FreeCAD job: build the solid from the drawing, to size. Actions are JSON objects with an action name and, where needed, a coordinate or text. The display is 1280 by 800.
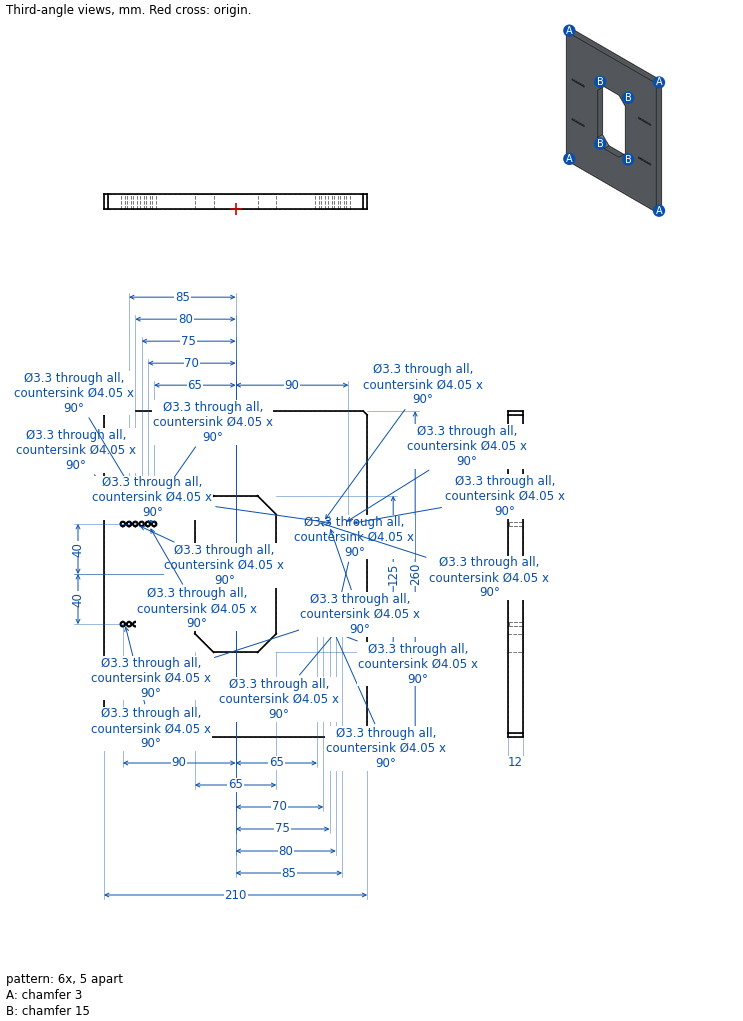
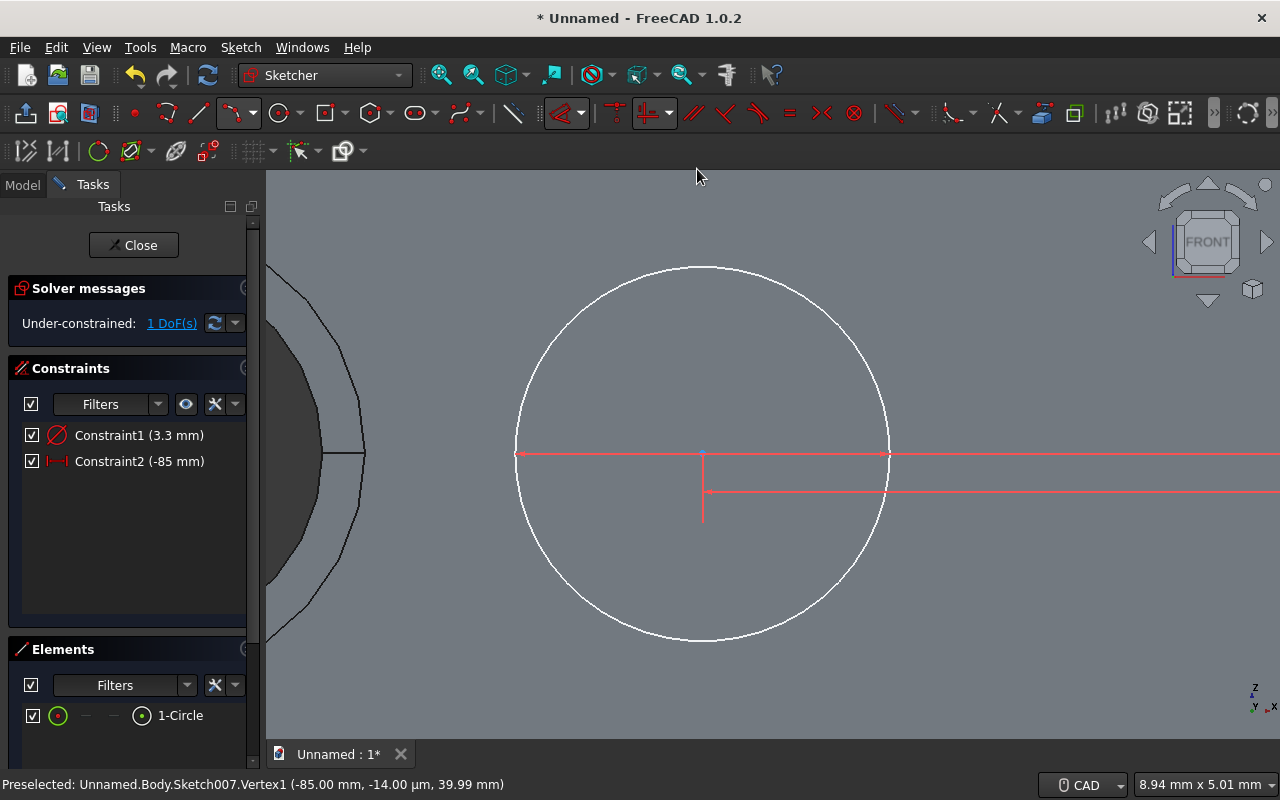
{"action": "left_click", "coordinate": [703, 454]}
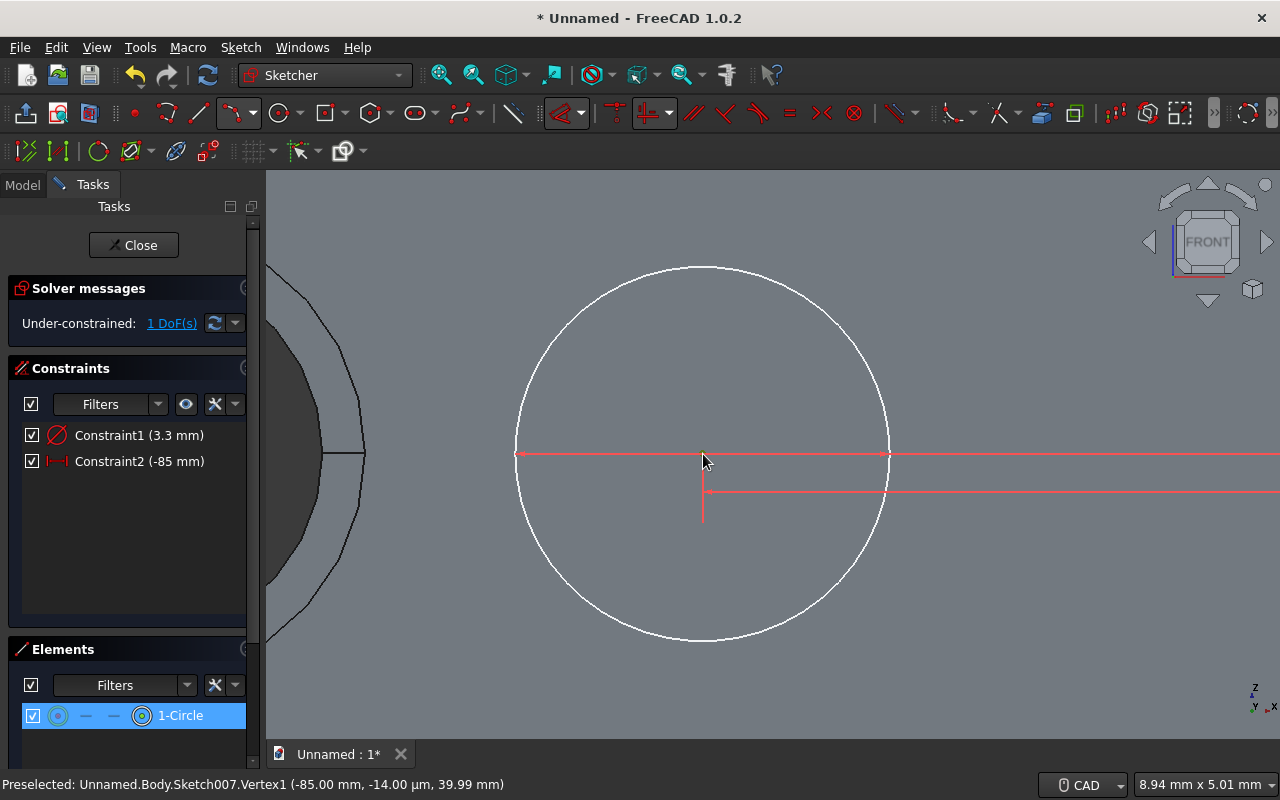
{"action": "key", "text": "i"}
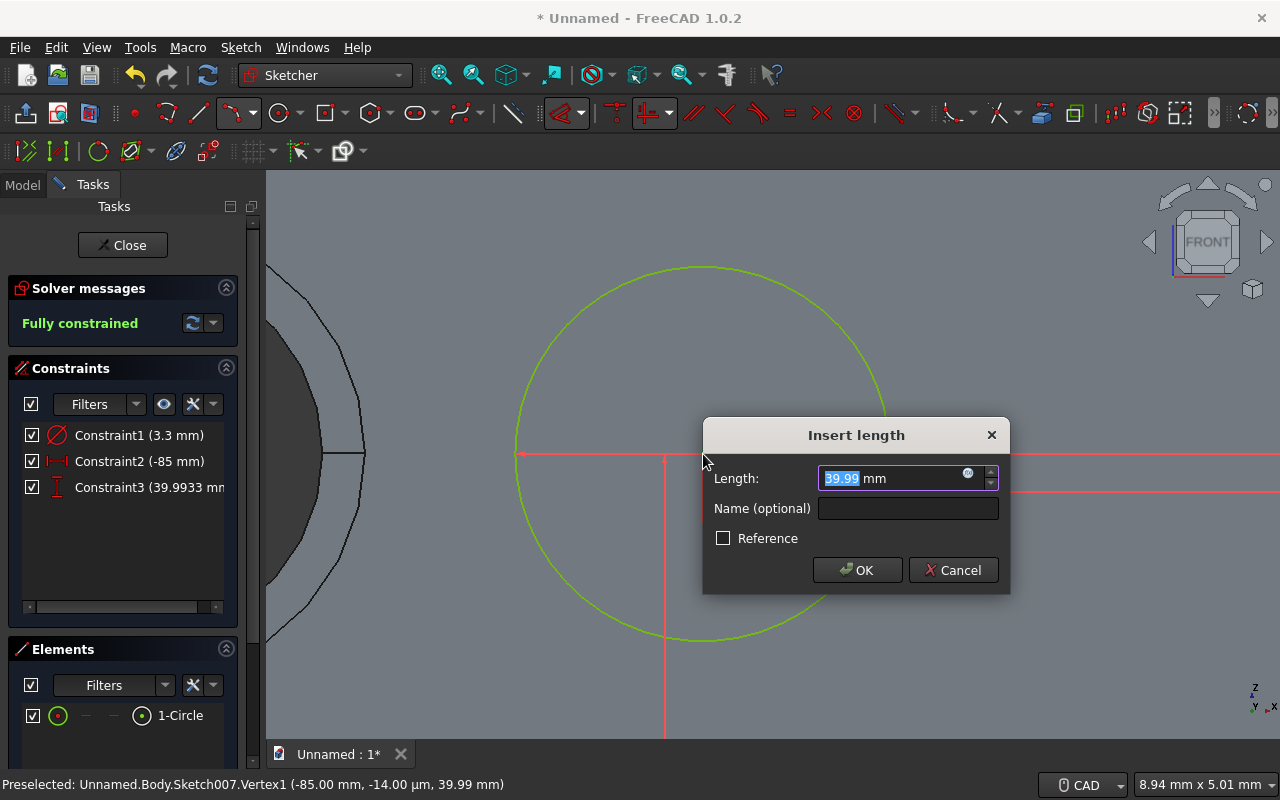
{"action": "type", "text": "40"}
{"action": "key", "text": "Return"}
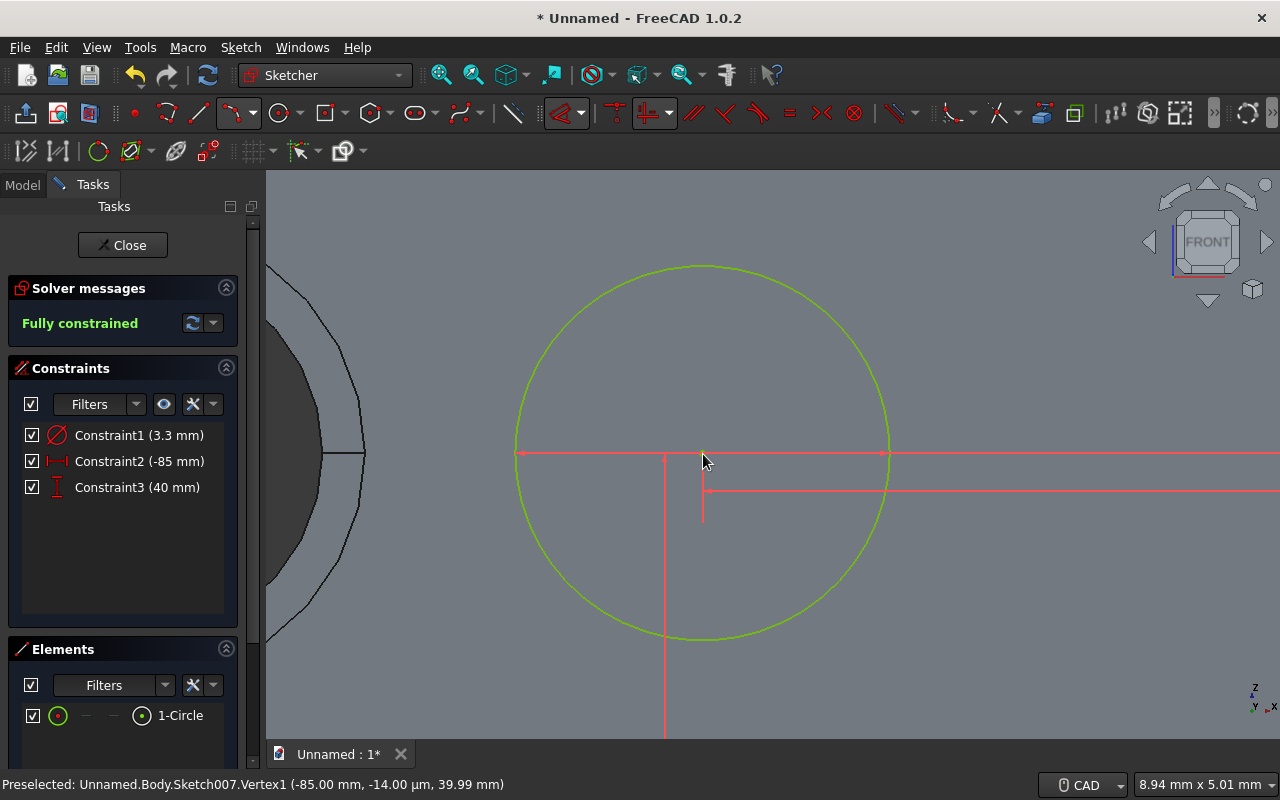
{"action": "left_click", "coordinate": [123, 245]}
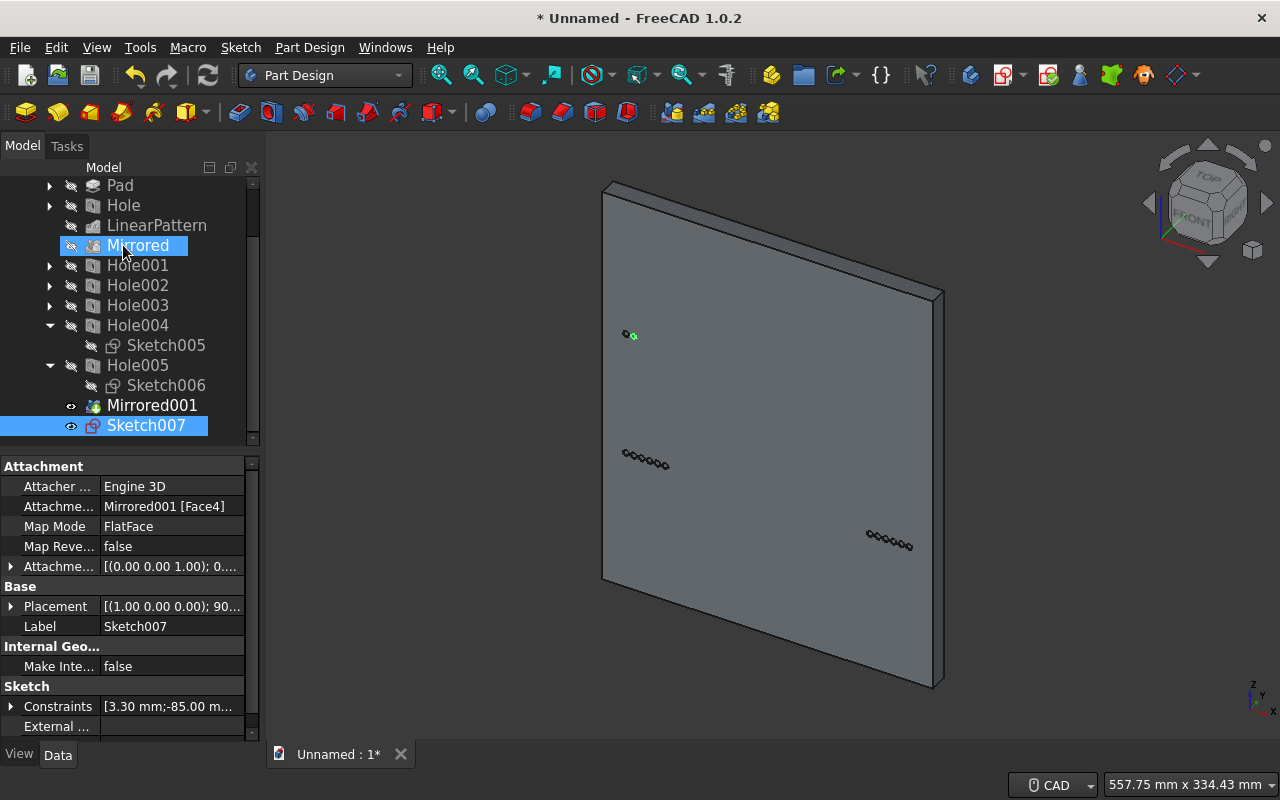
{"action": "left_click", "coordinate": [272, 112]}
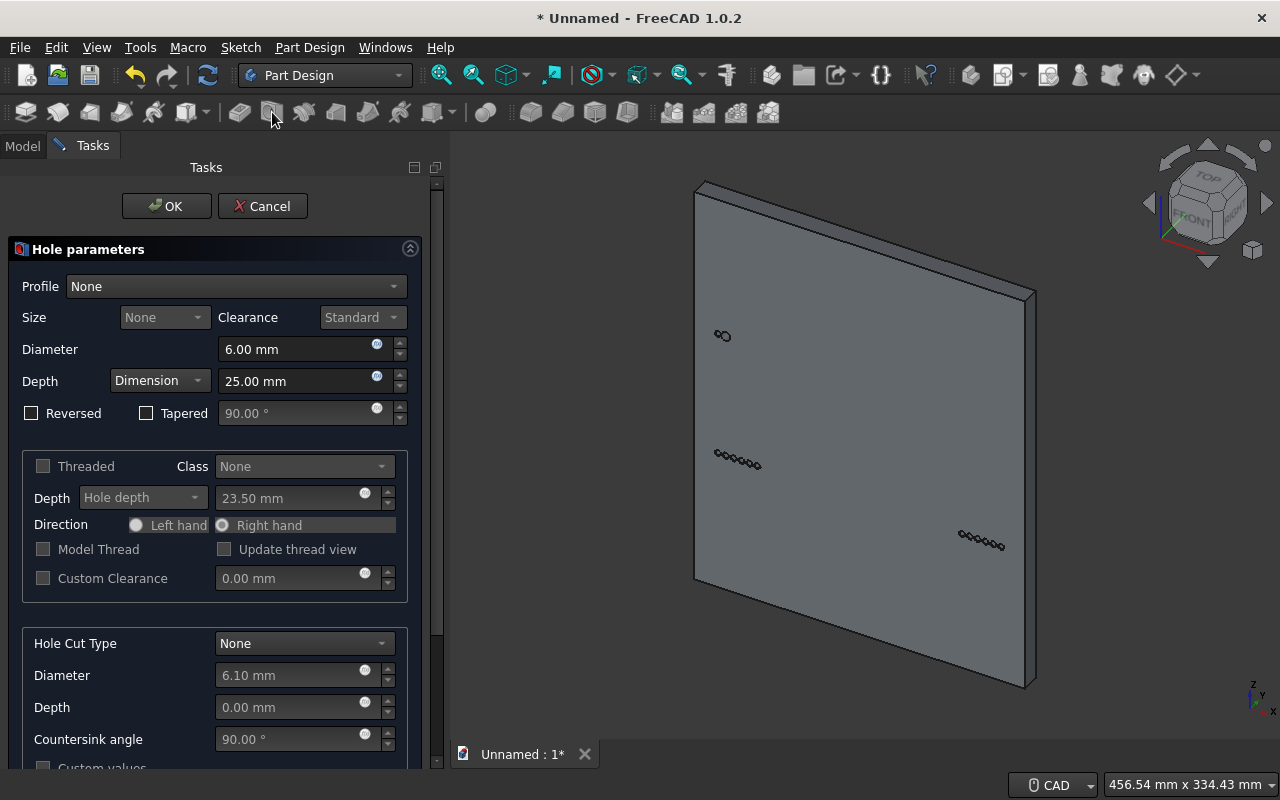
{"action": "triple_click", "coordinate": [305, 349]}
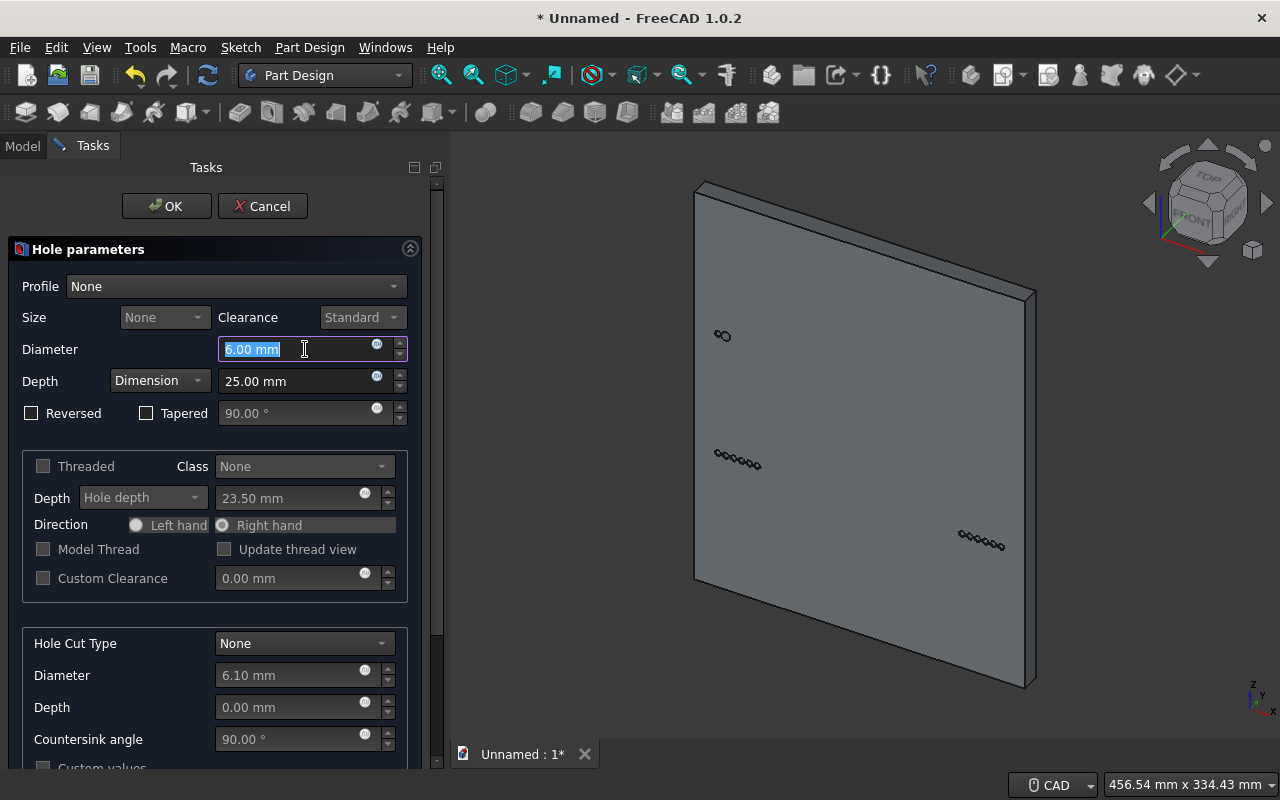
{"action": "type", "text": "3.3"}
{"action": "key", "text": "Tab"}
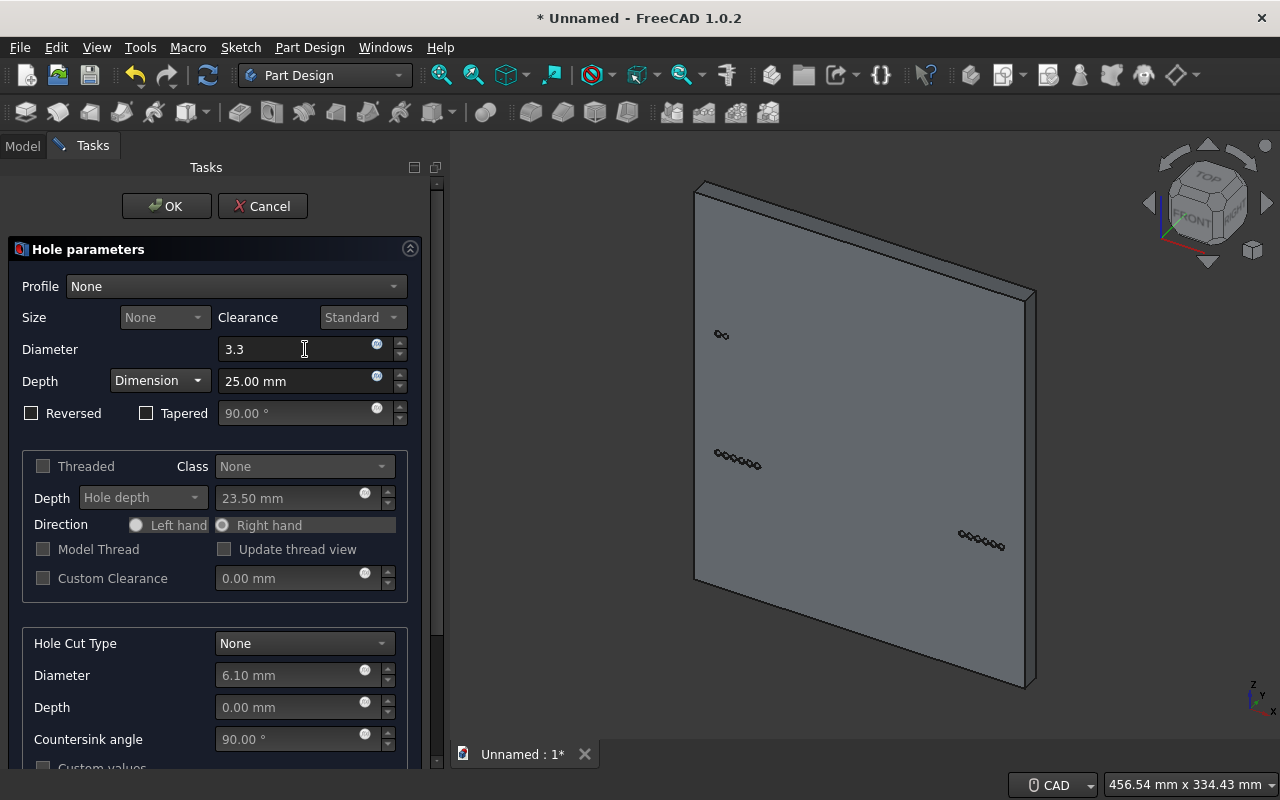
{"action": "left_click", "coordinate": [161, 380]}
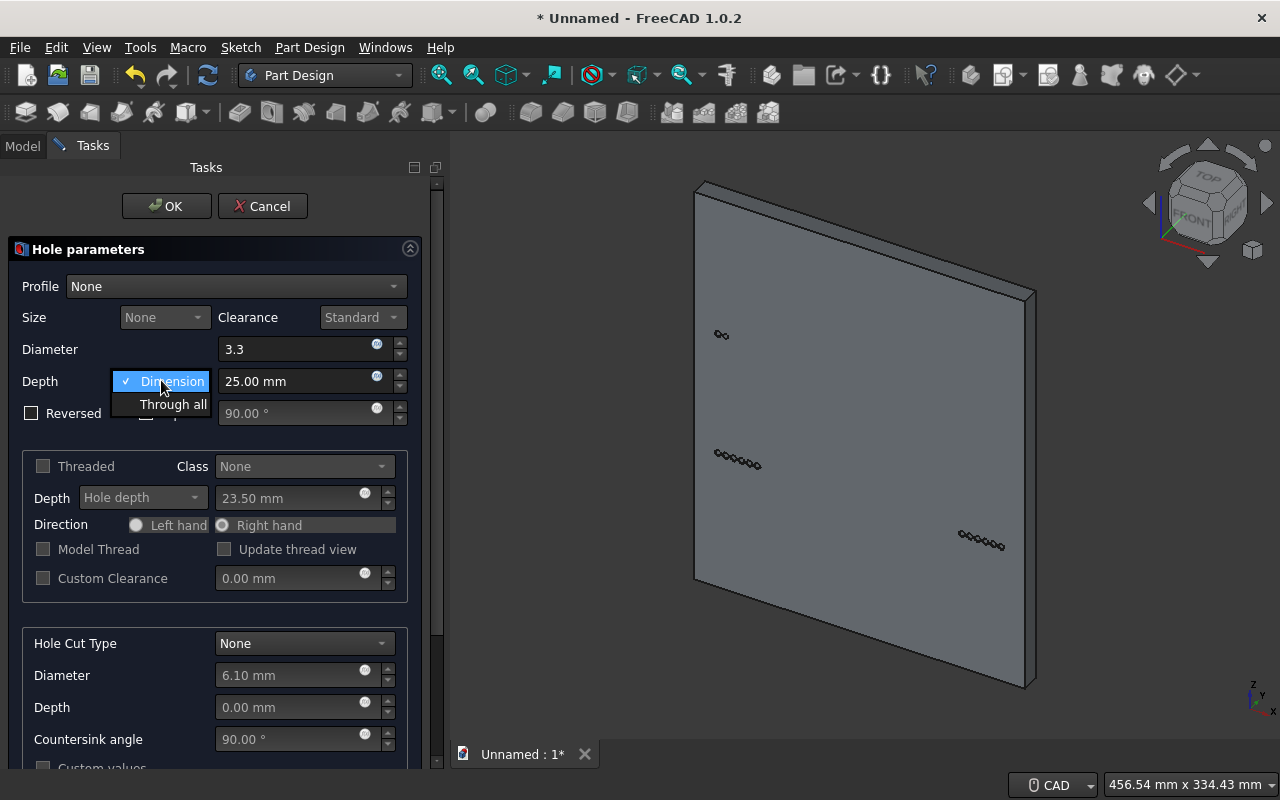
{"action": "left_click", "coordinate": [160, 404]}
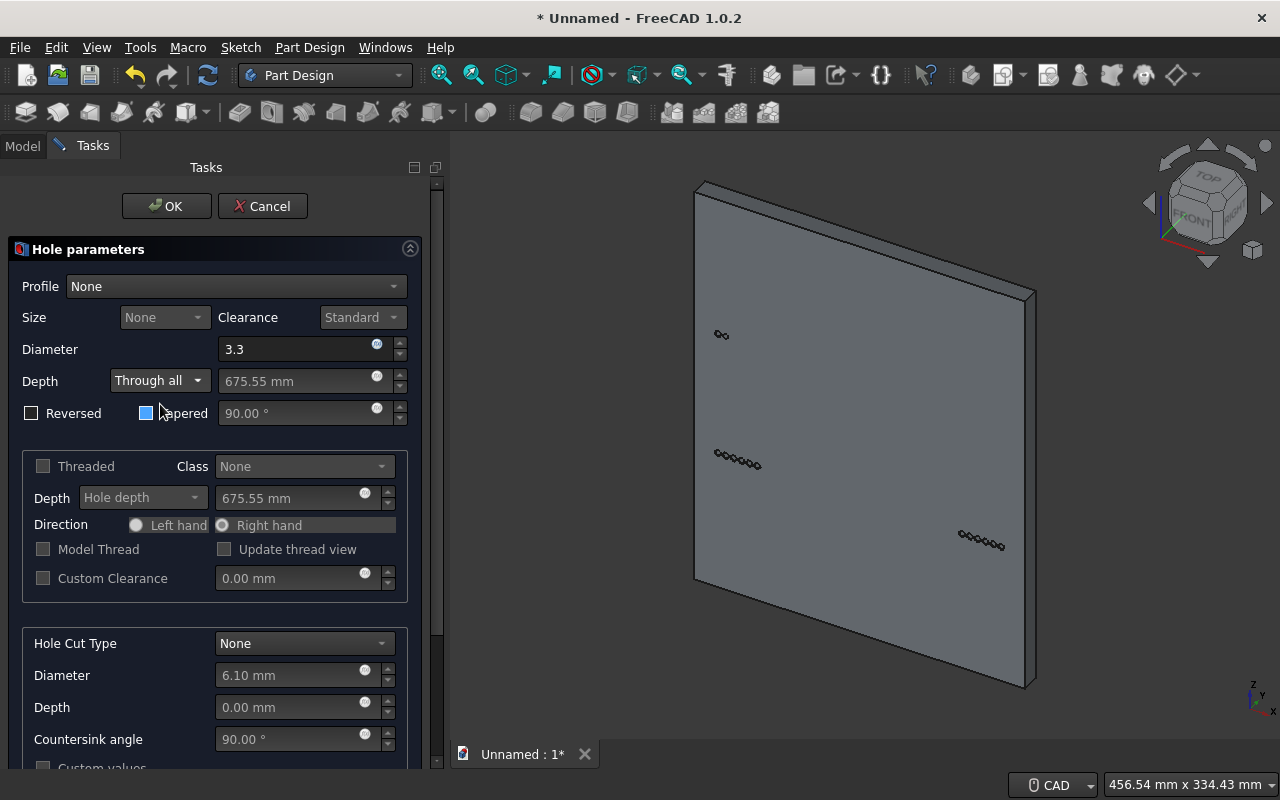
{"action": "left_click", "coordinate": [306, 644]}